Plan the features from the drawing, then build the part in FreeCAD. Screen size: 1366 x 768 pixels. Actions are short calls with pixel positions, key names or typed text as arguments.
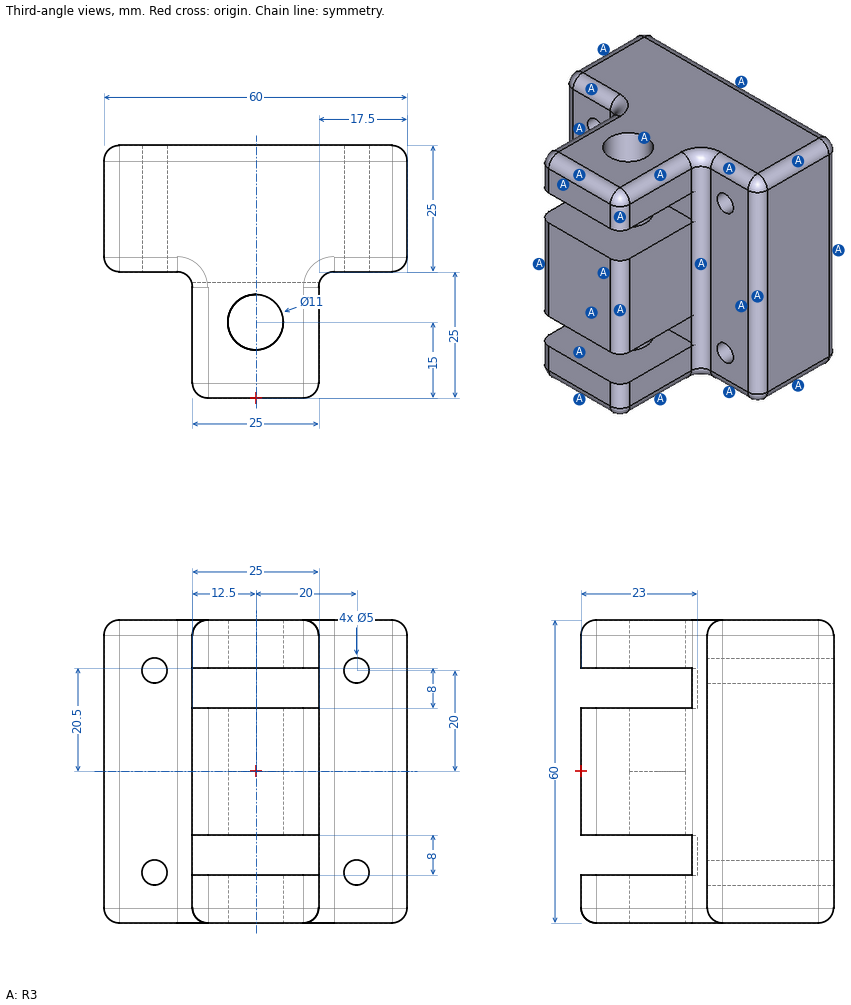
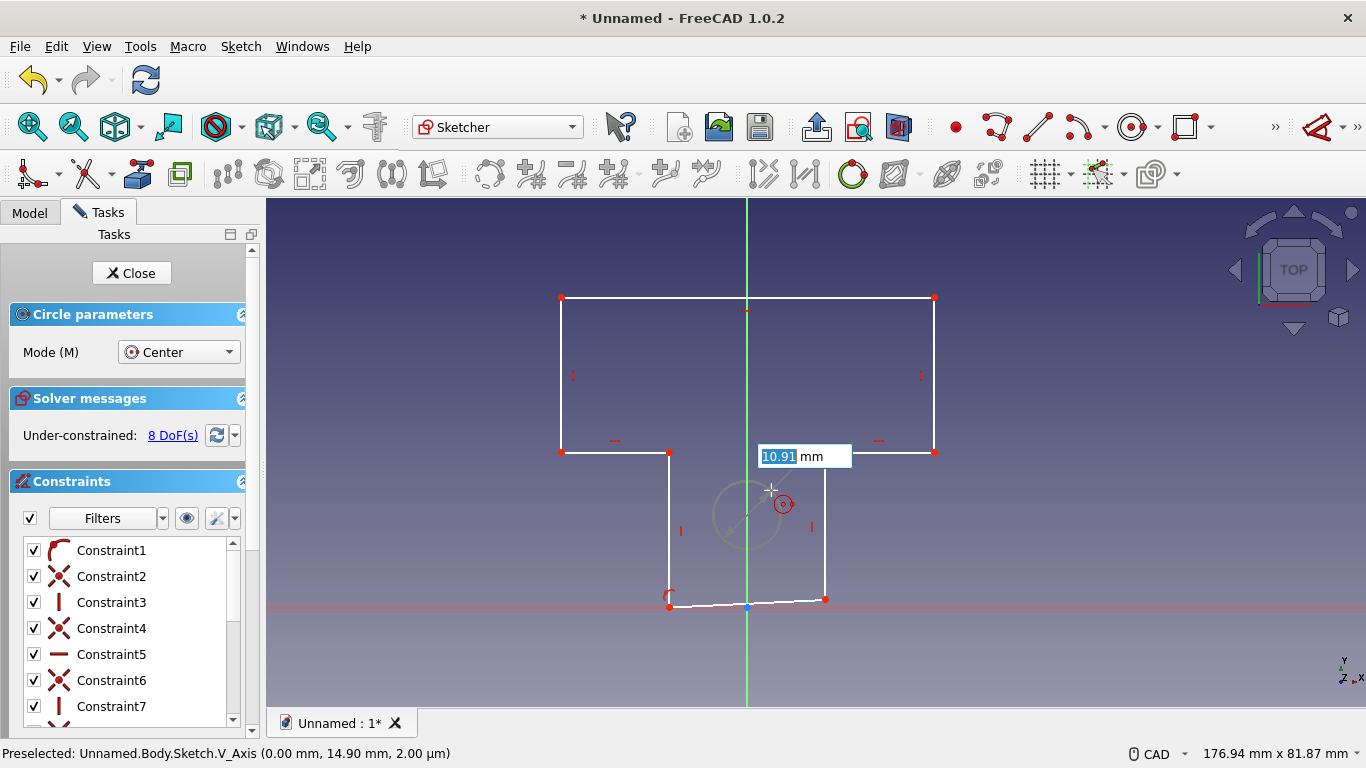
text(11)
key(Return)
key(Escape)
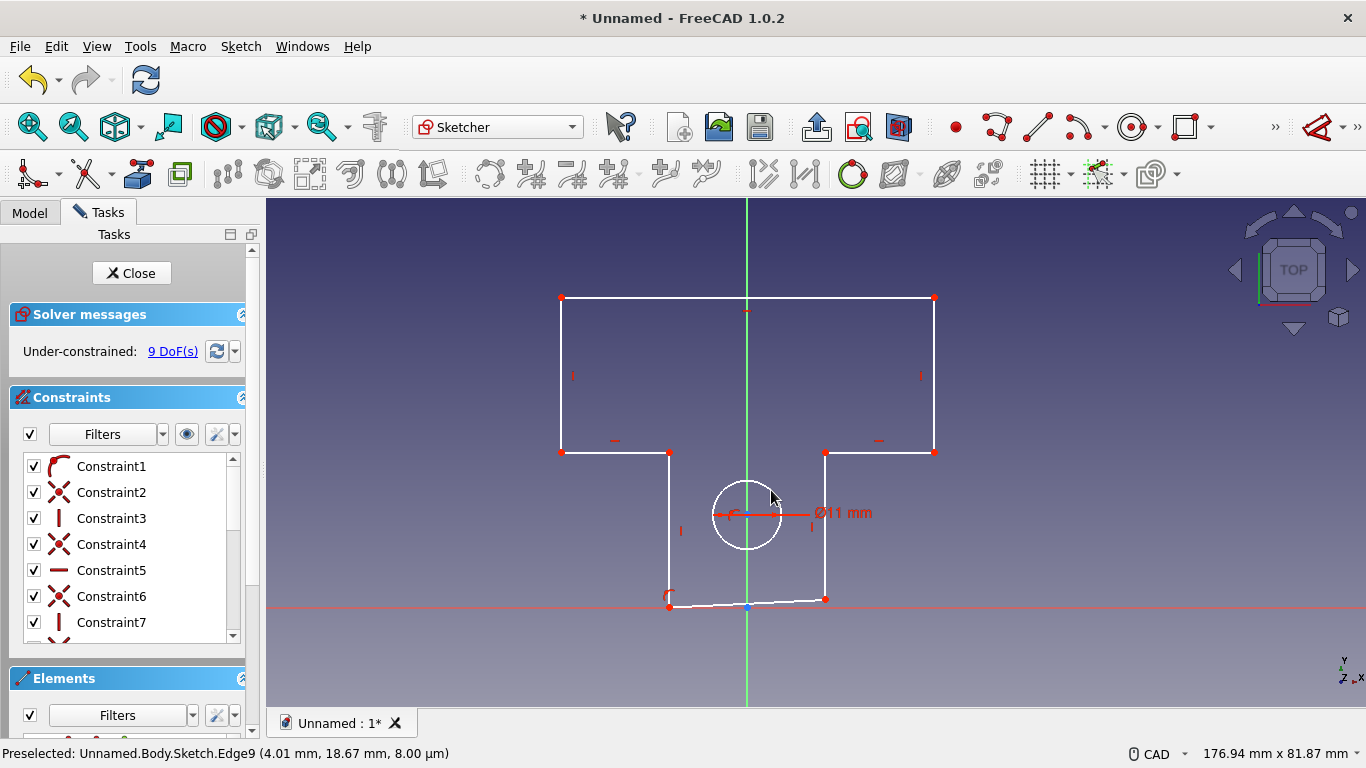
click(716, 605)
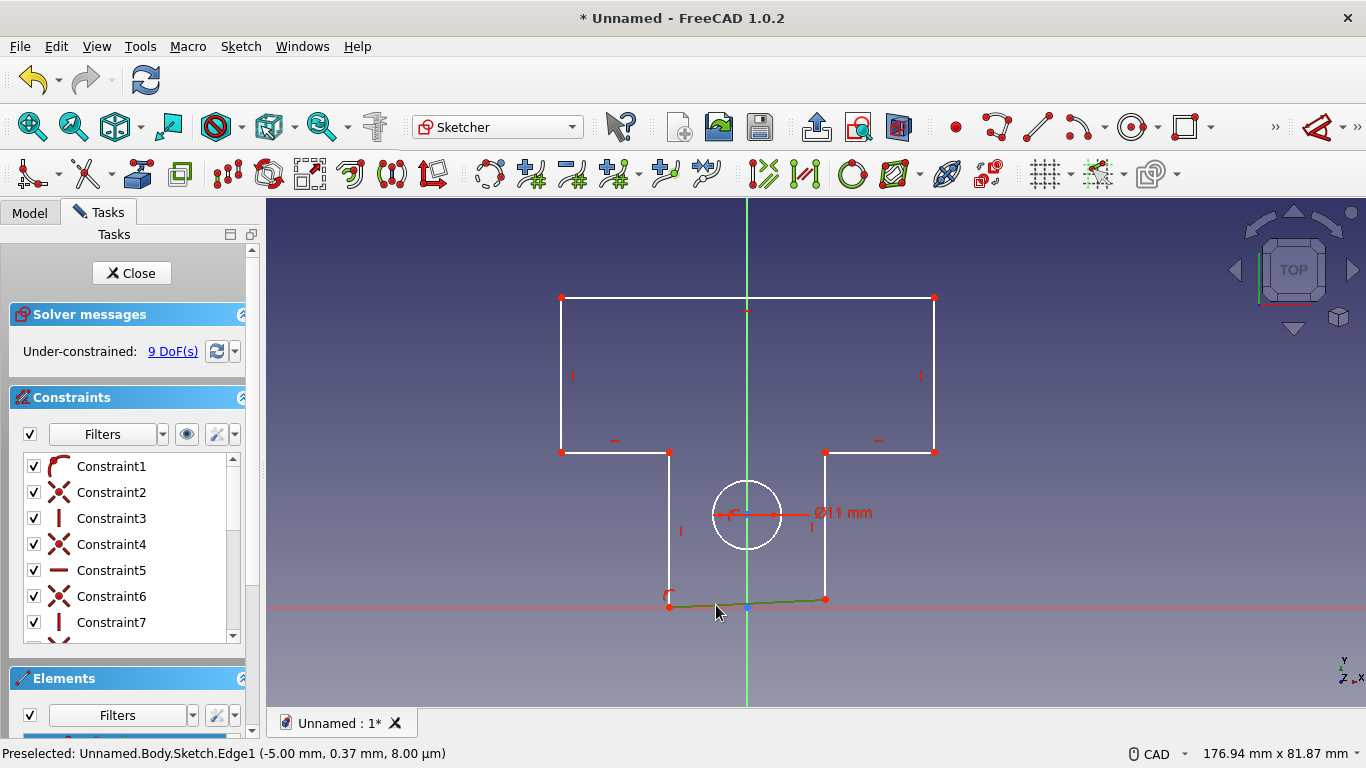
key(h)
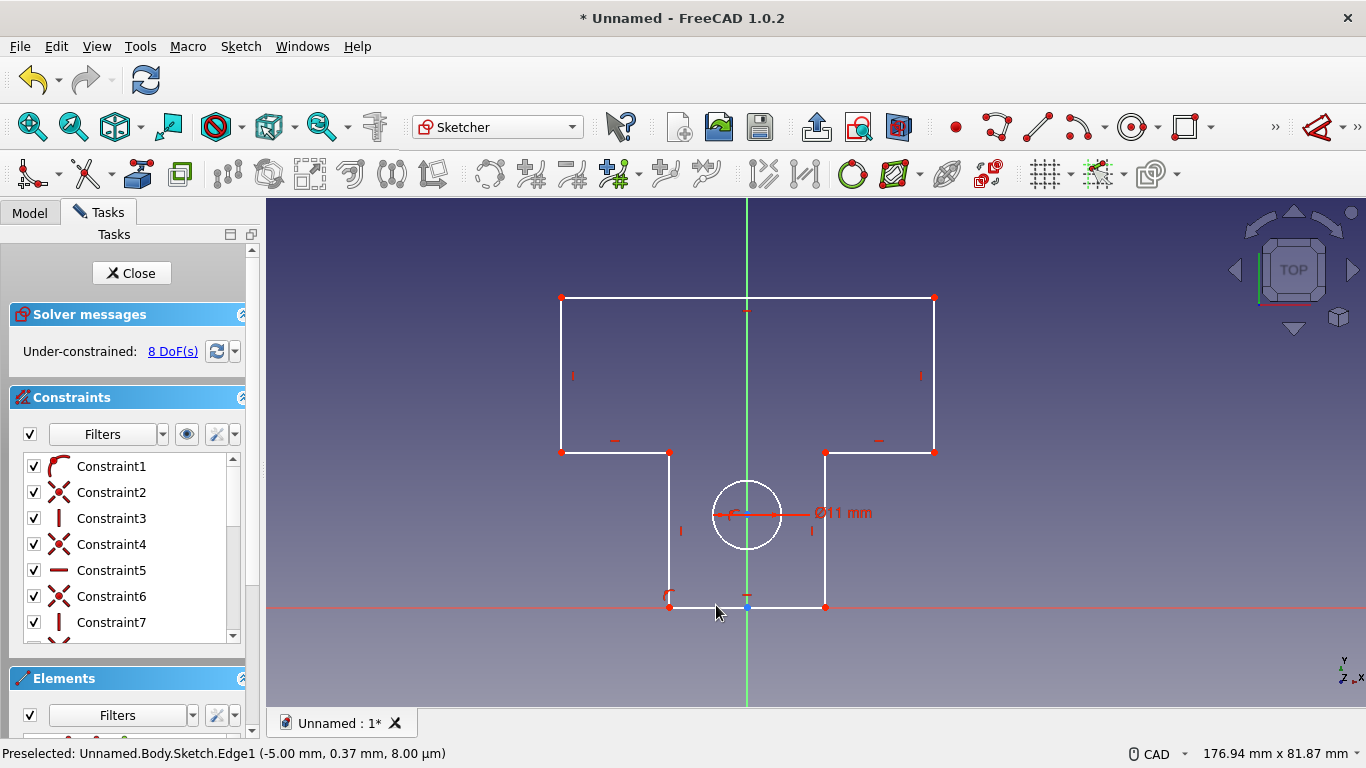
click(934, 453)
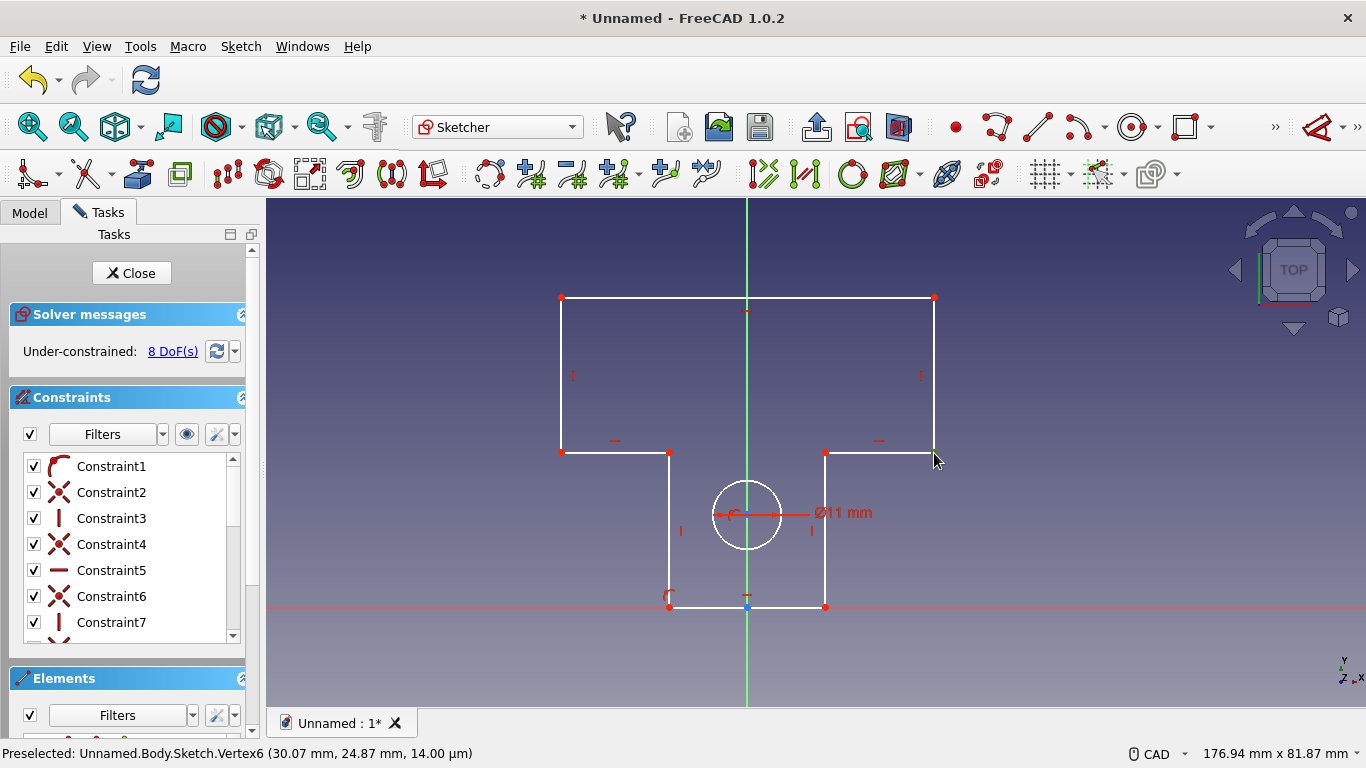
click(561, 453)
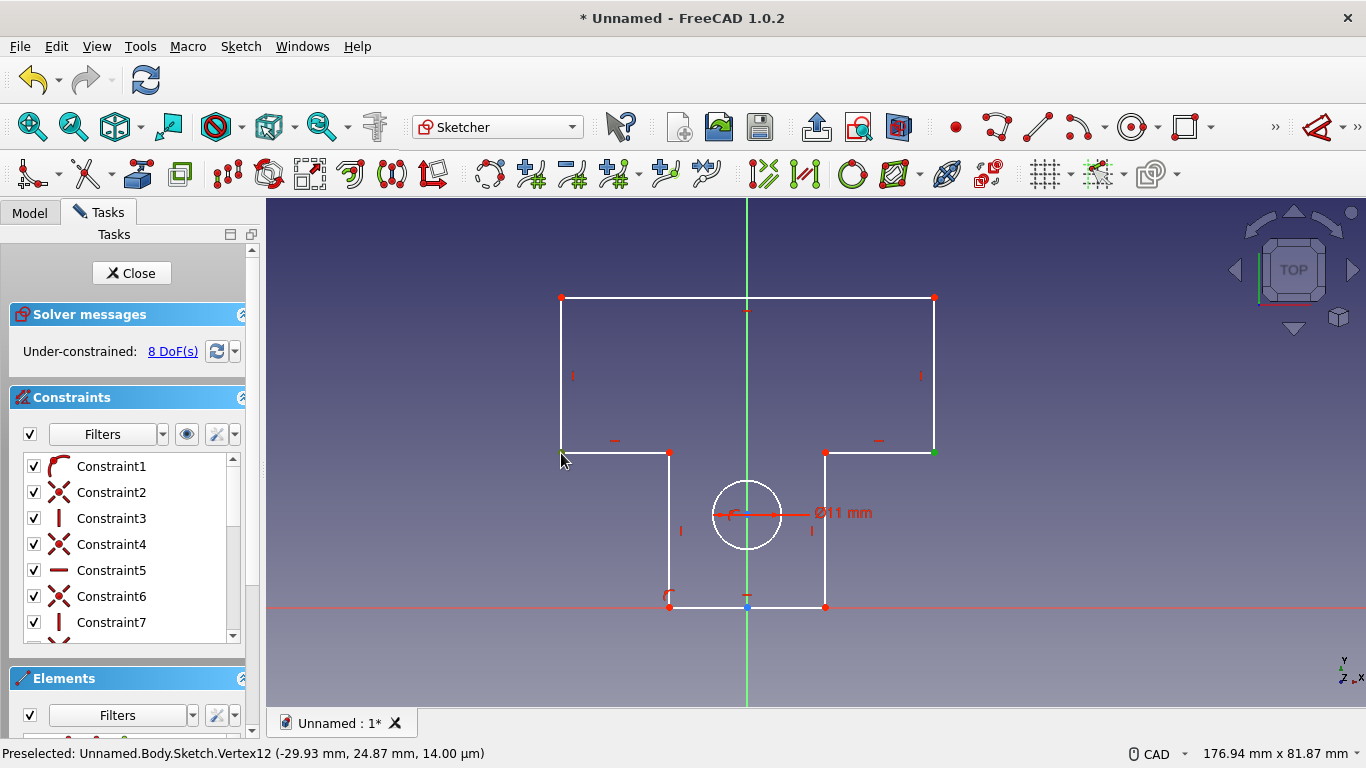
click(747, 647)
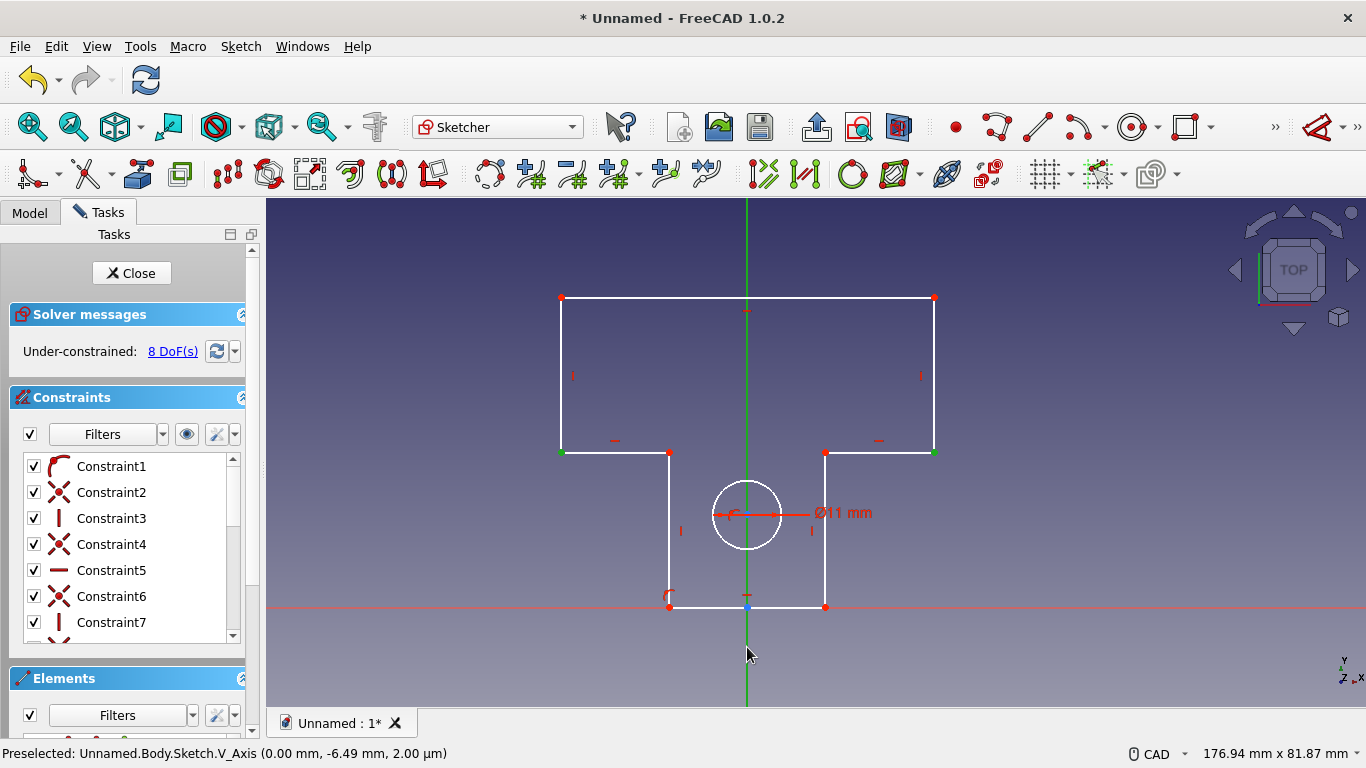
key(s)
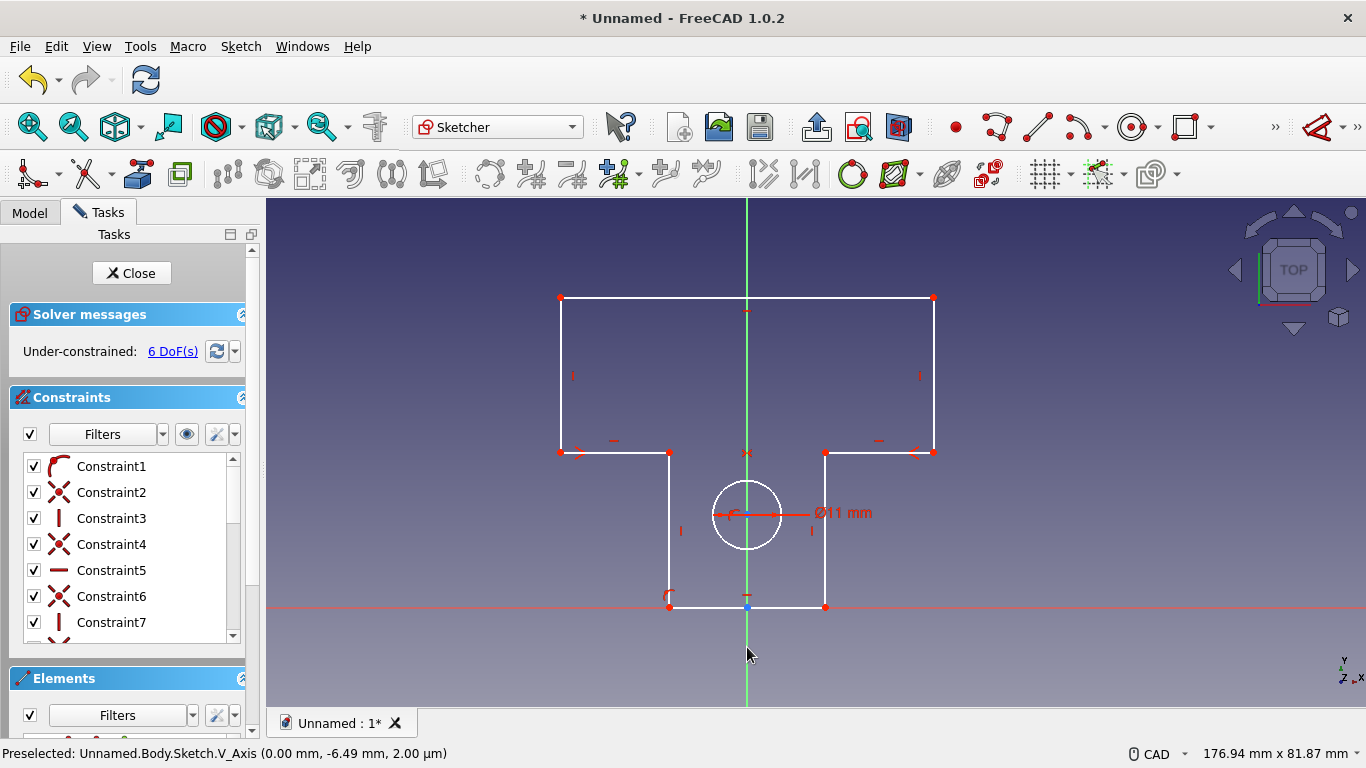
click(716, 608)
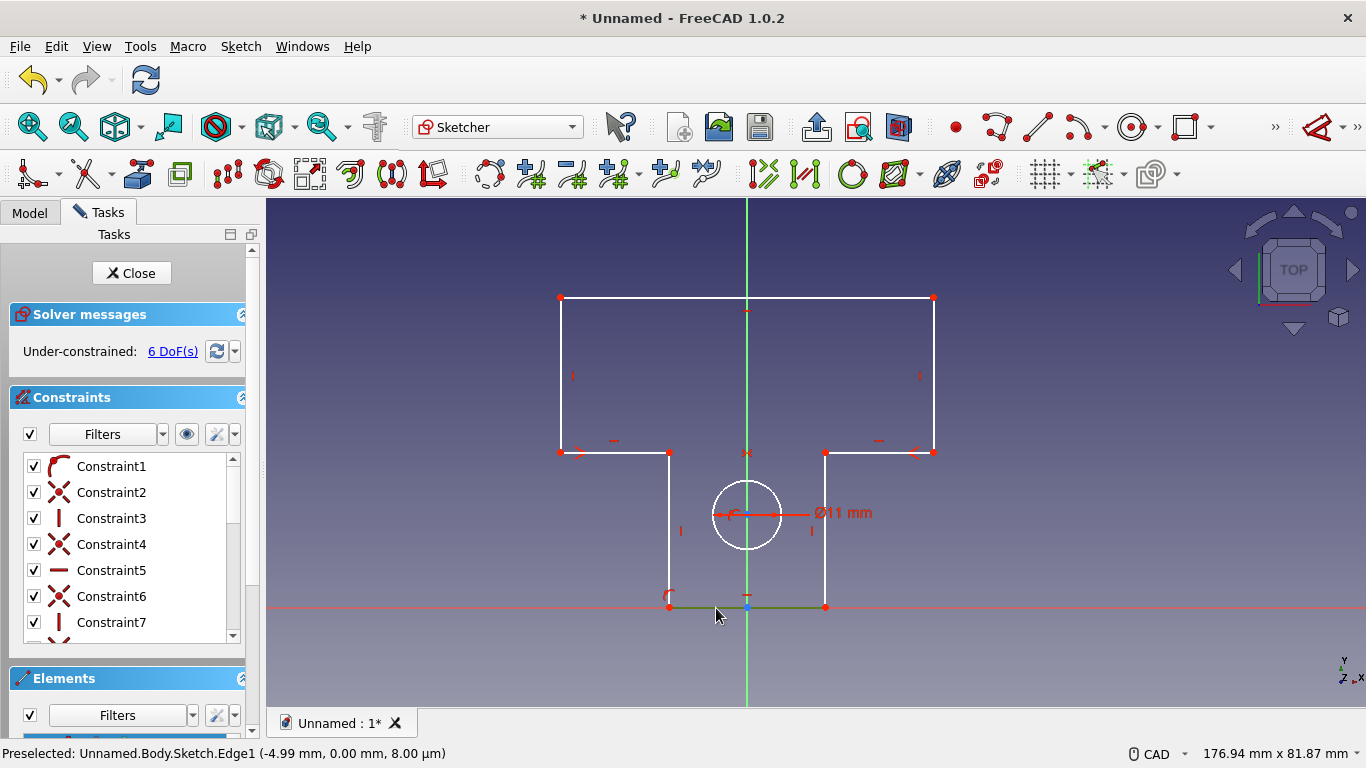
key(l)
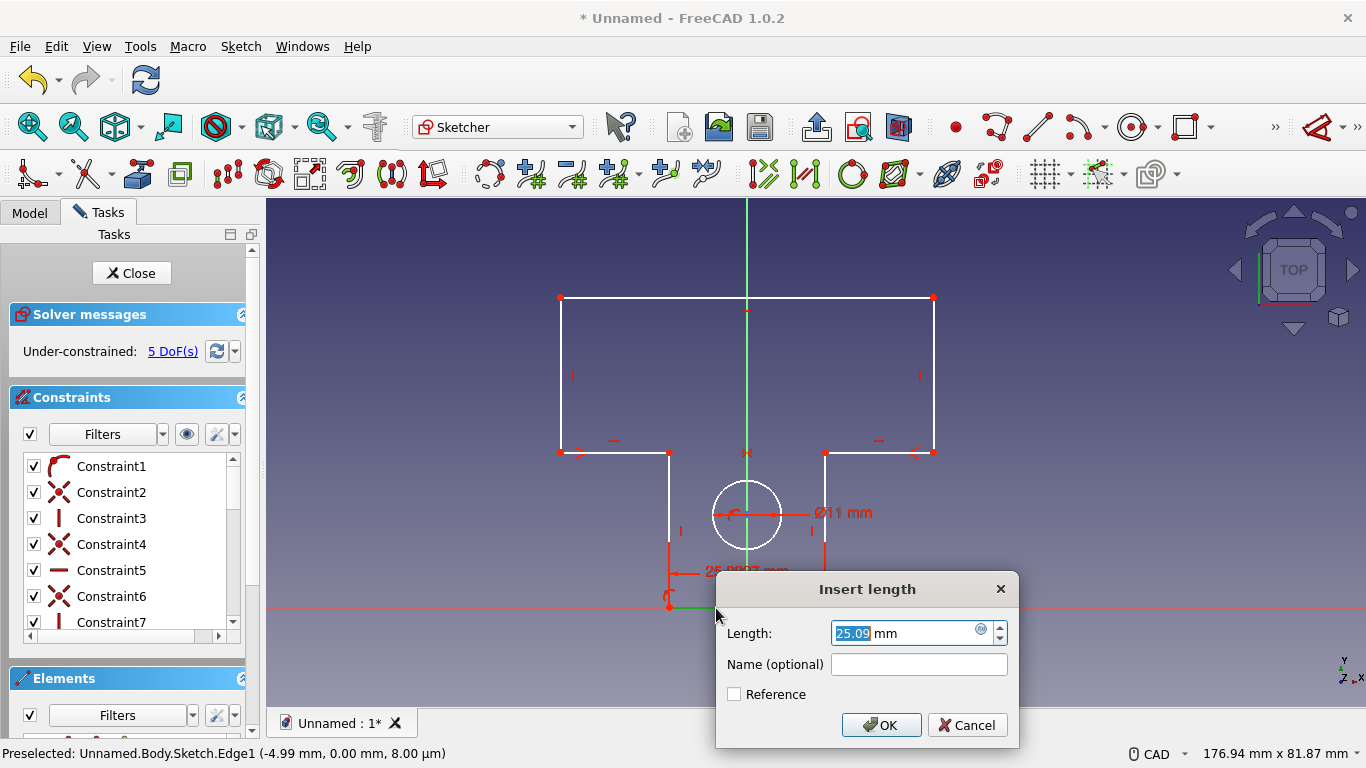
text(25)
key(Return)